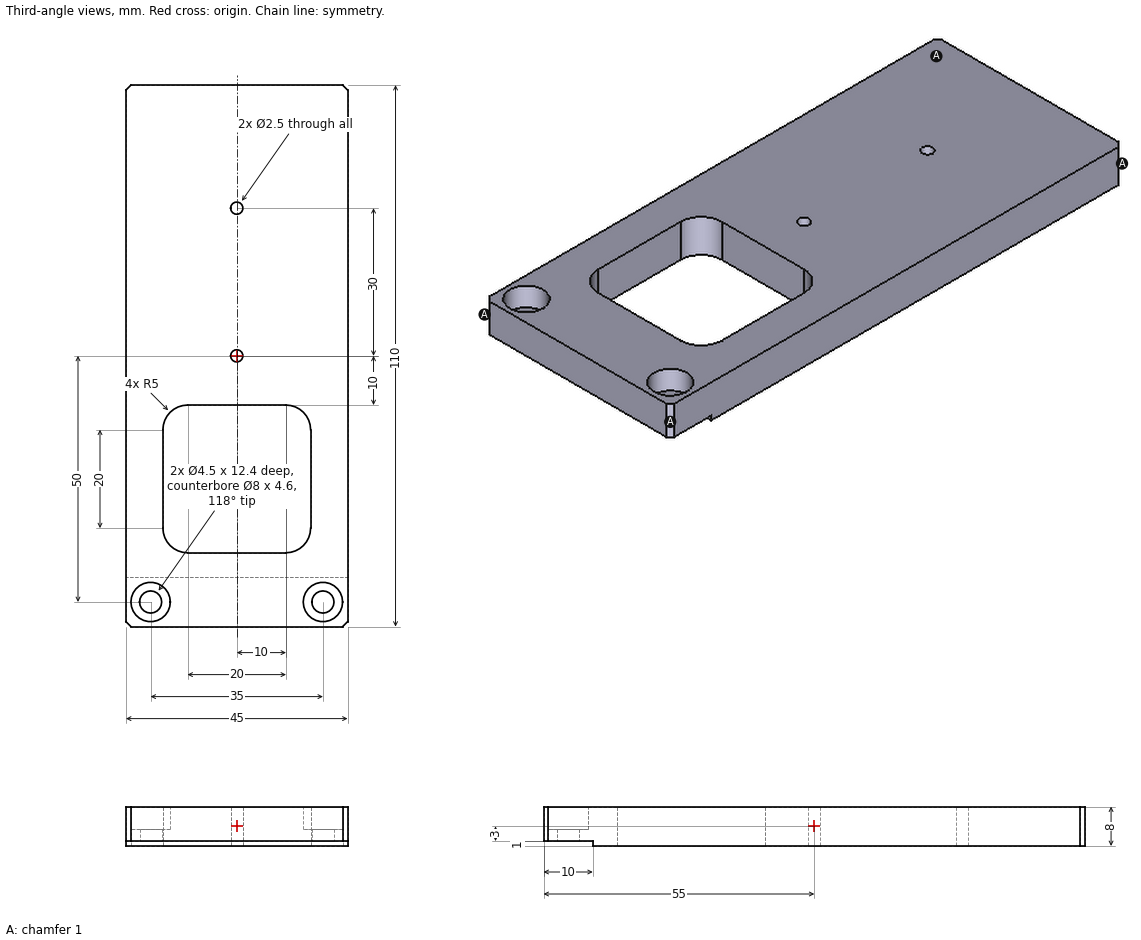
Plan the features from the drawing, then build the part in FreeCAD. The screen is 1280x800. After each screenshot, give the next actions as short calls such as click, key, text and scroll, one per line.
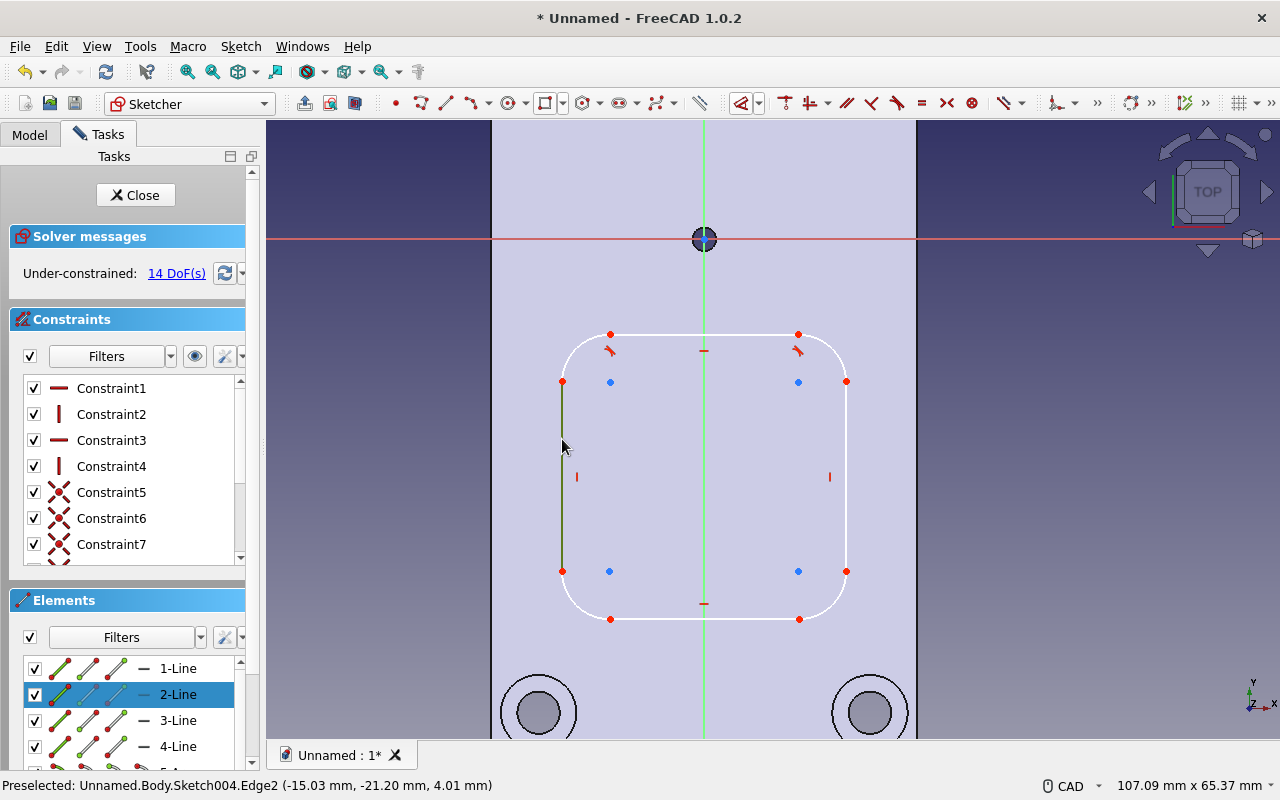
click(588, 340)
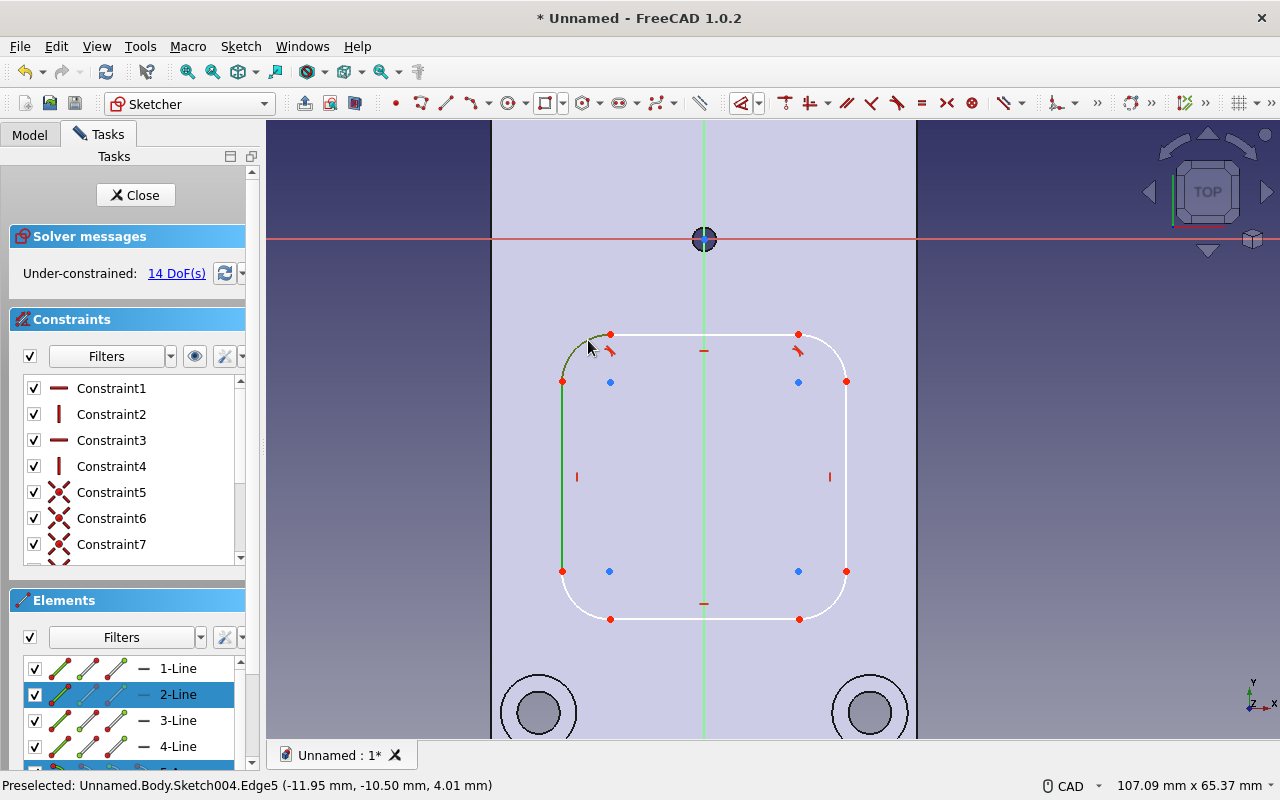
click(897, 104)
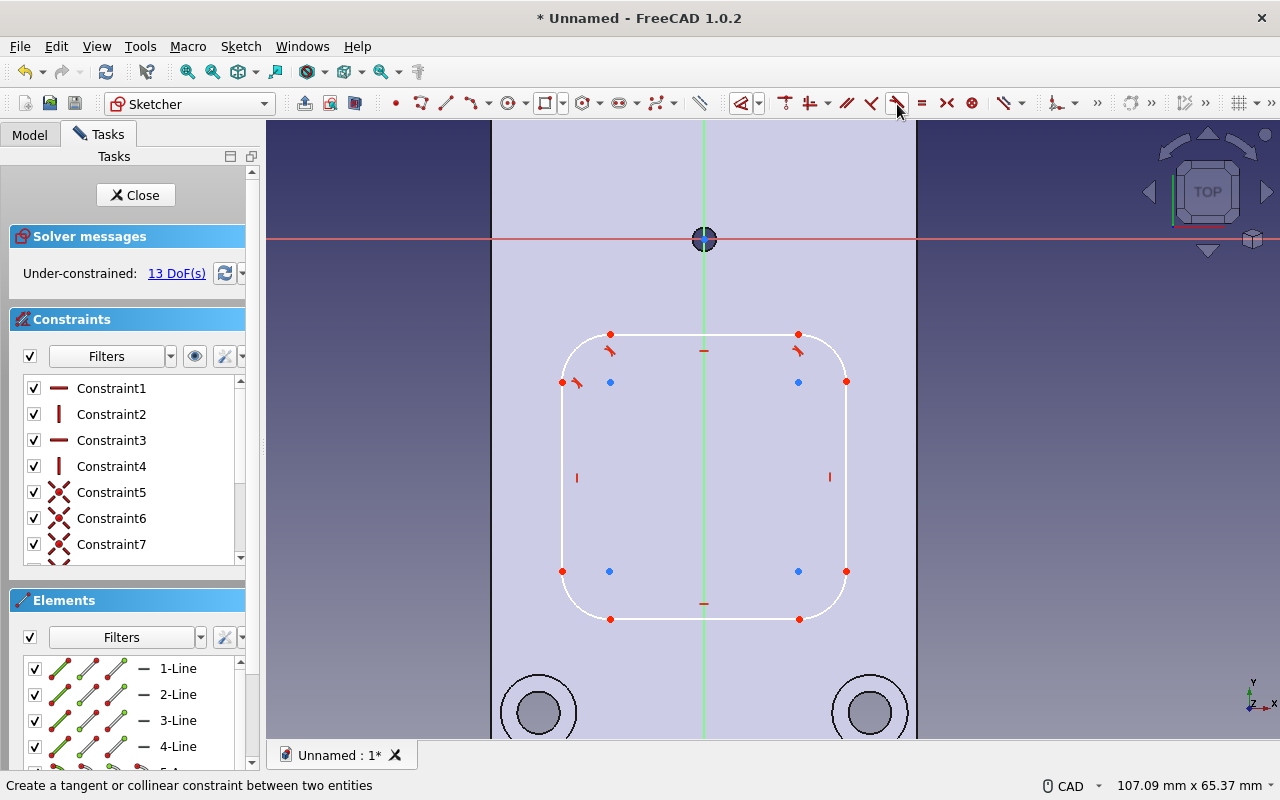
click(562, 440)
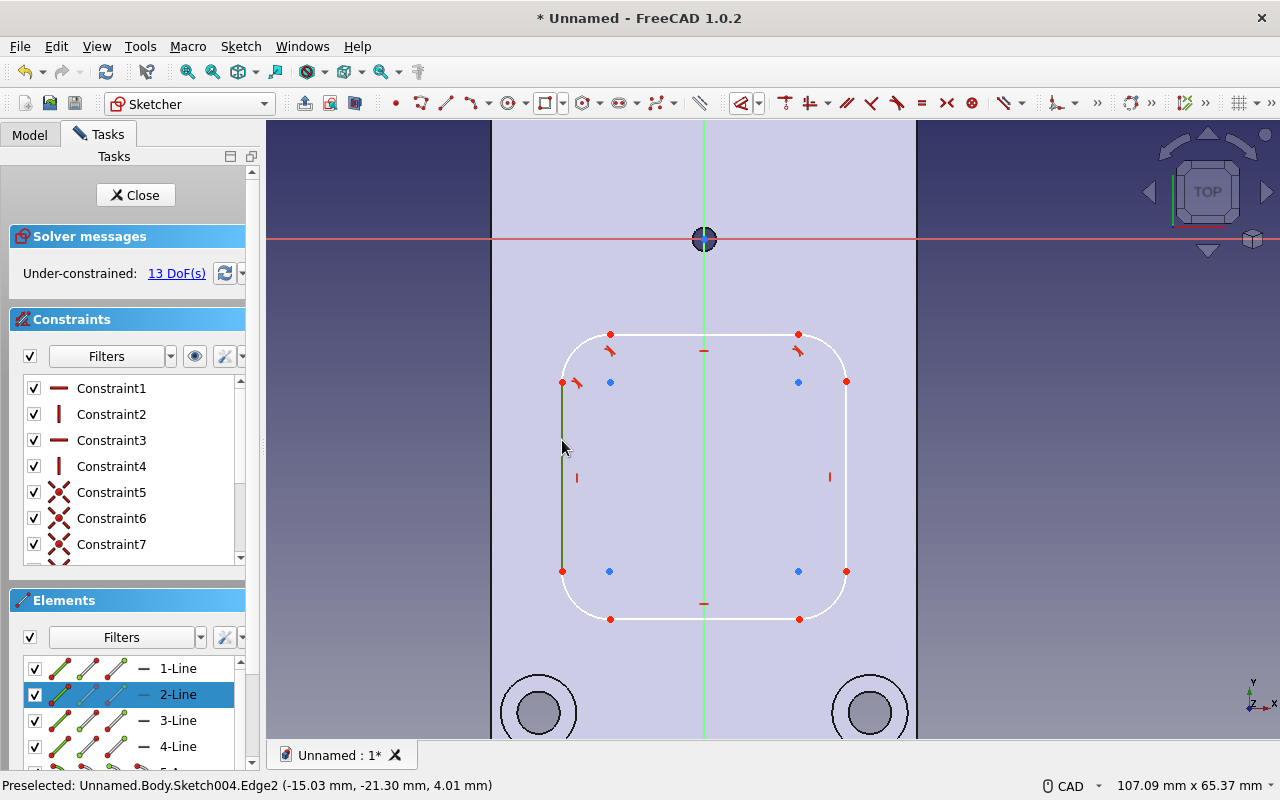
click(567, 593)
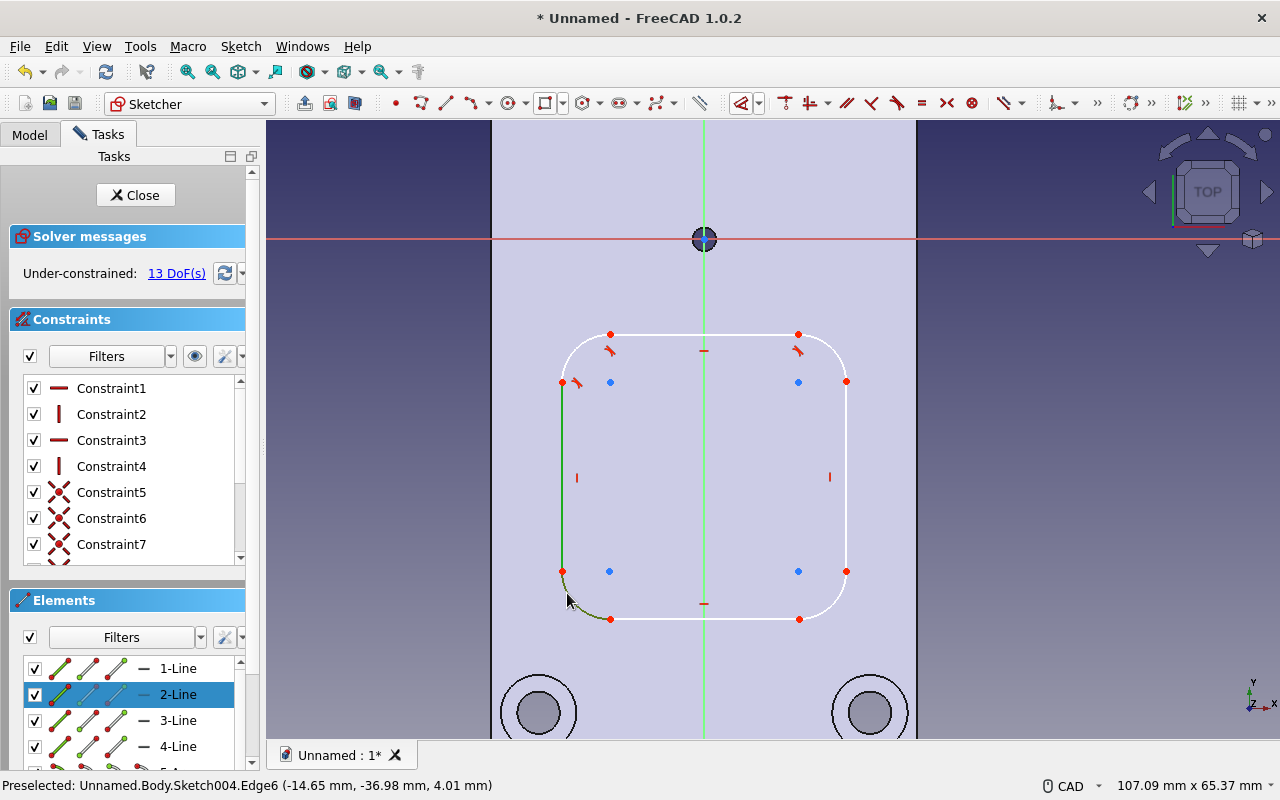
click(897, 104)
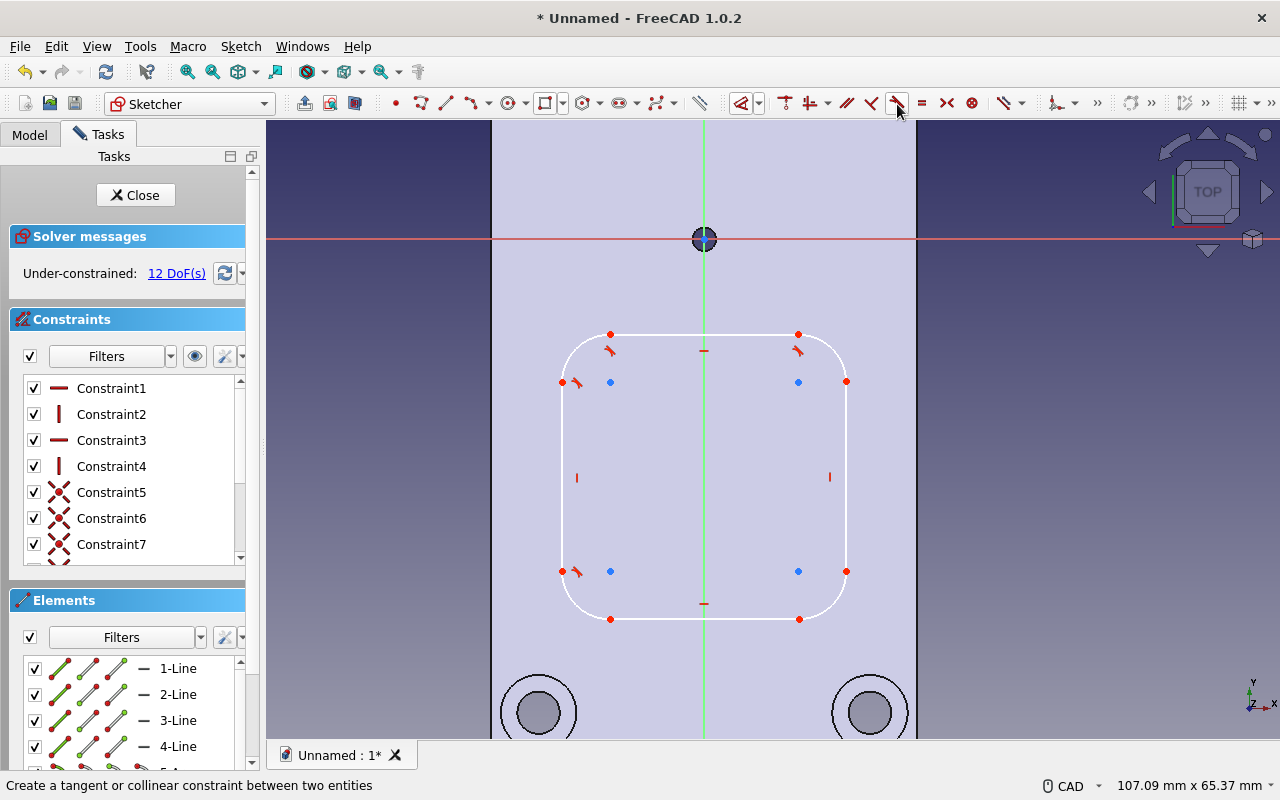
click(667, 619)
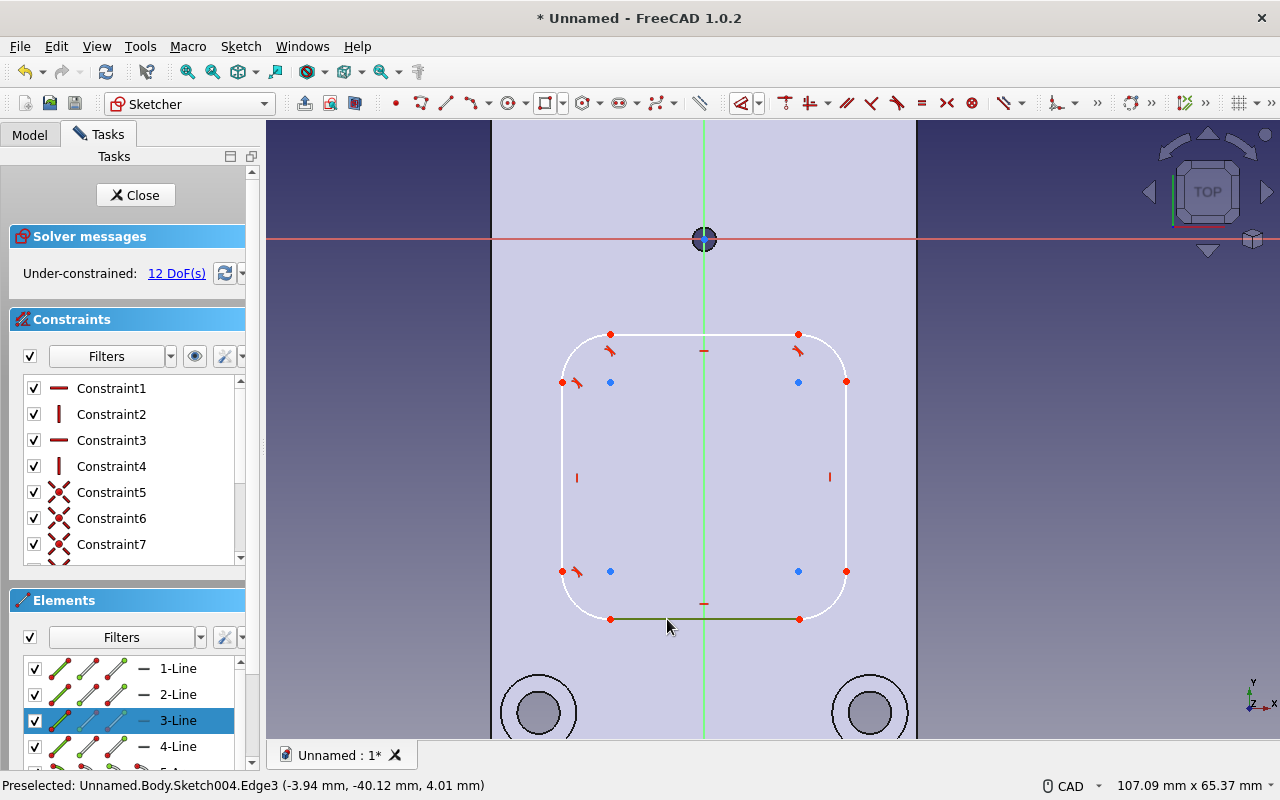
click(567, 593)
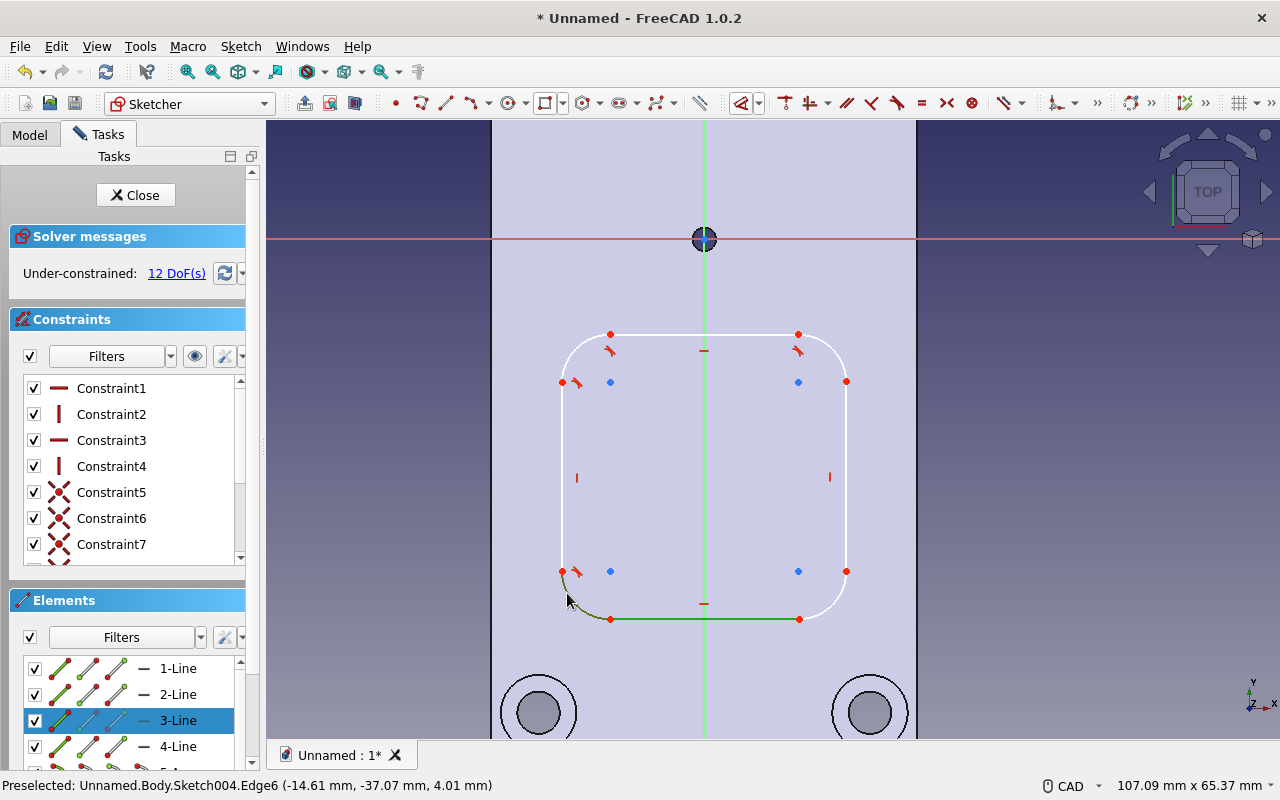
click(897, 104)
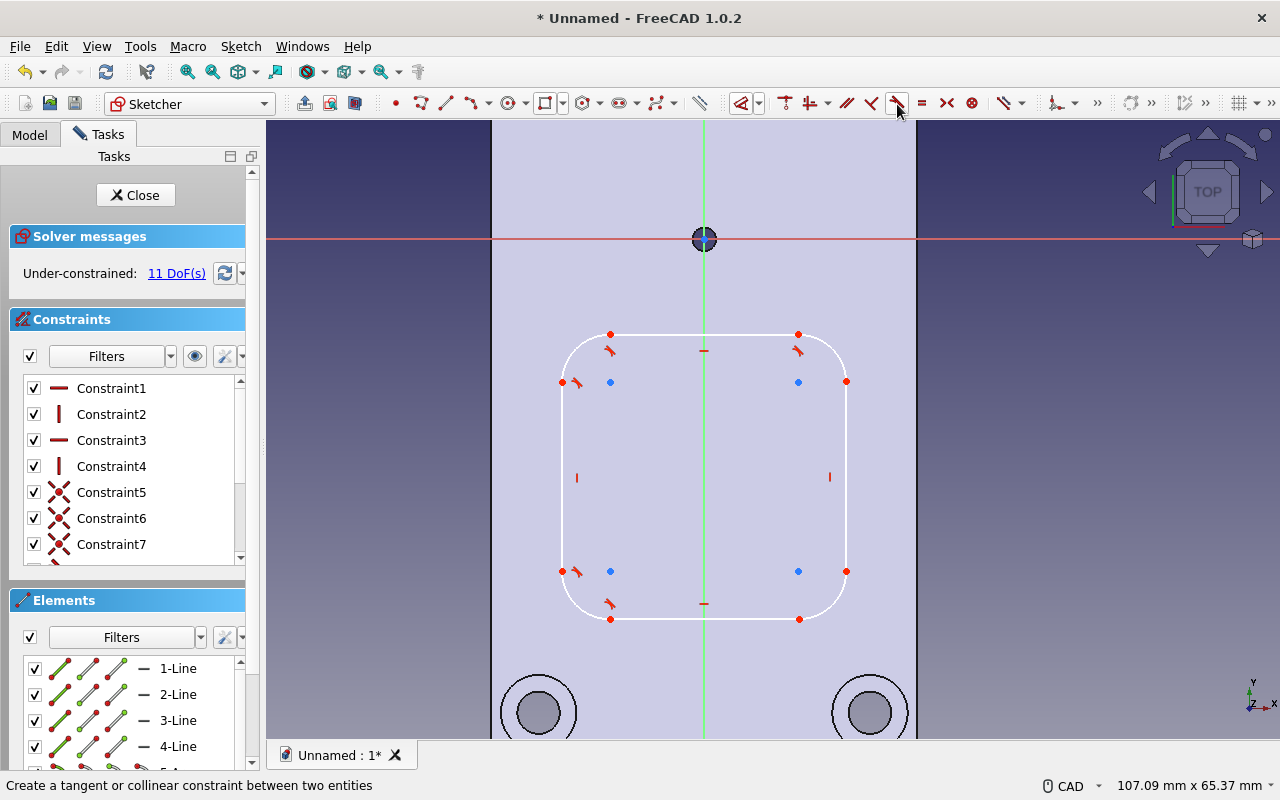
click(667, 619)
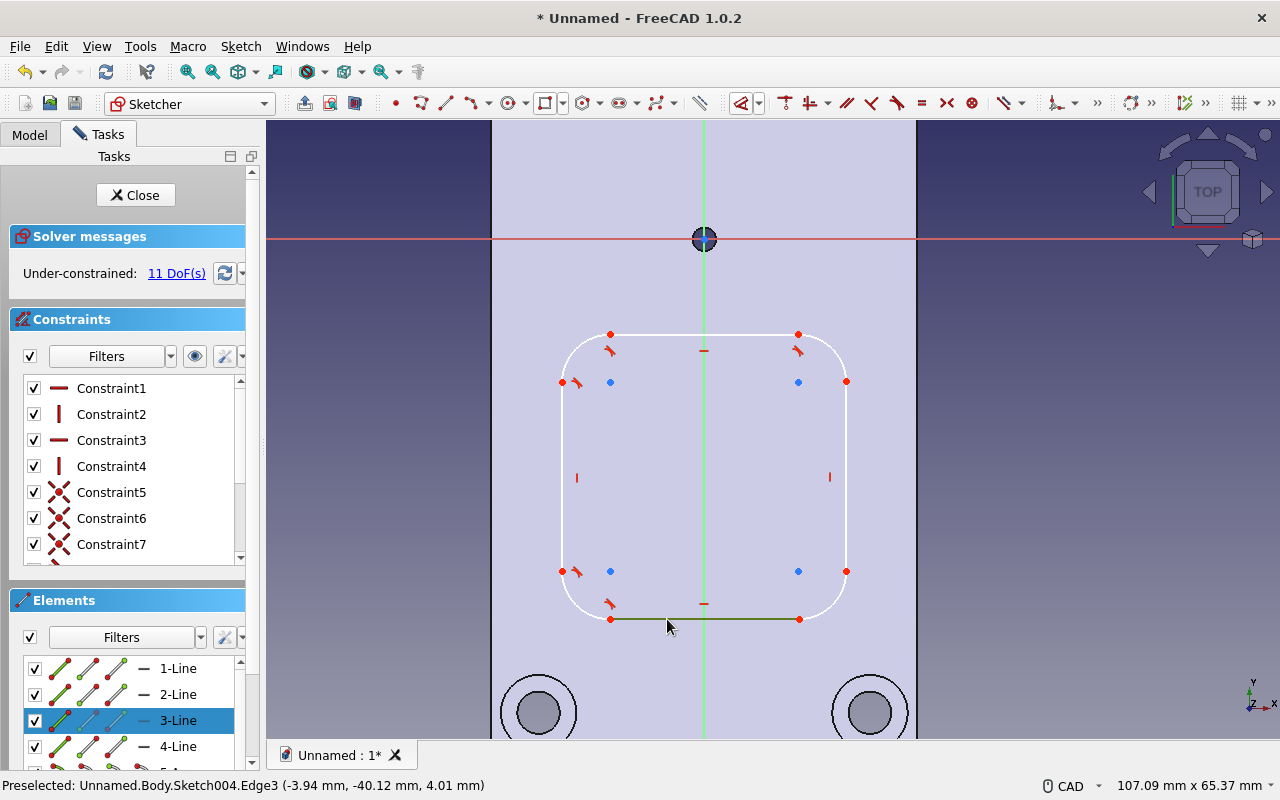
click(820, 614)